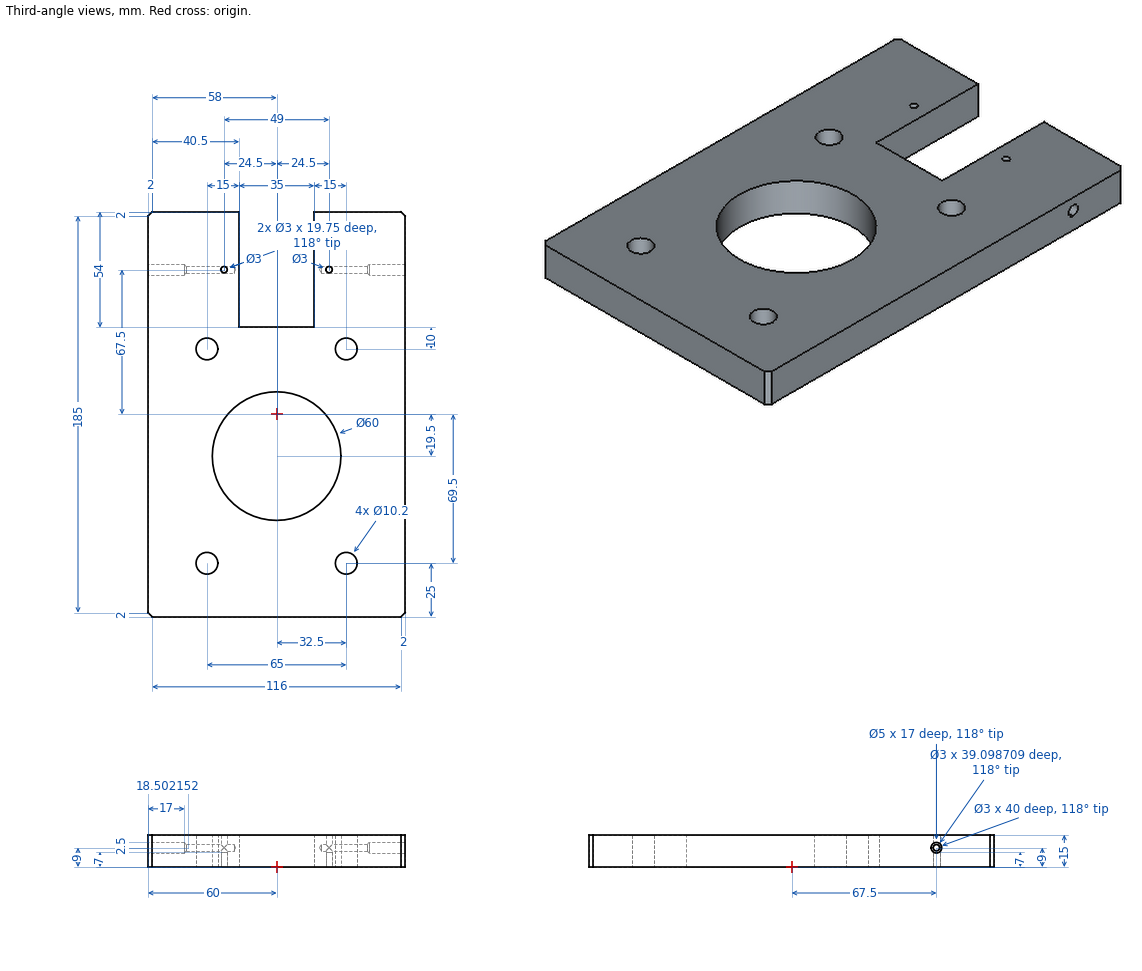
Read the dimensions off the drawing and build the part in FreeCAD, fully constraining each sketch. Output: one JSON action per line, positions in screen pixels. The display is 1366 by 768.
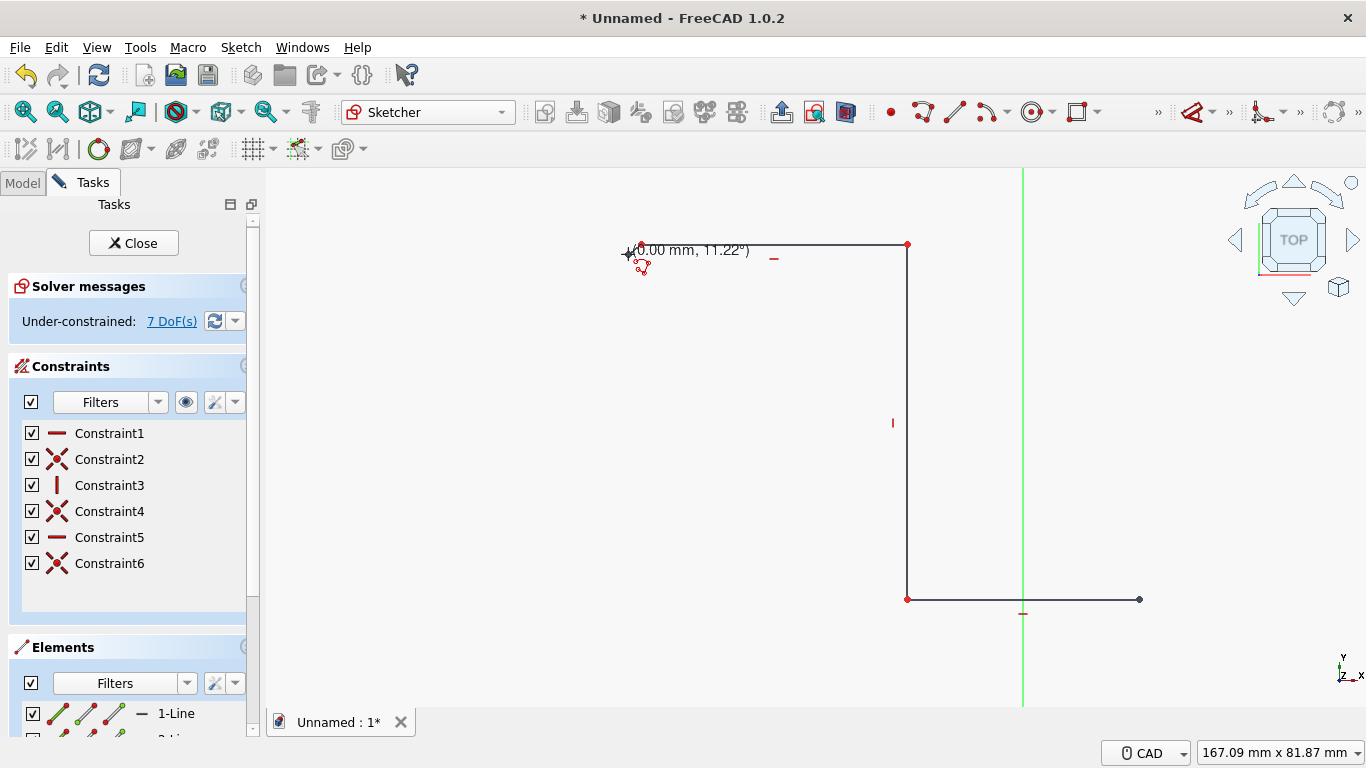
{"action": "scroll", "coordinate": [629, 254], "scroll_direction": "down", "scroll_amount": 6}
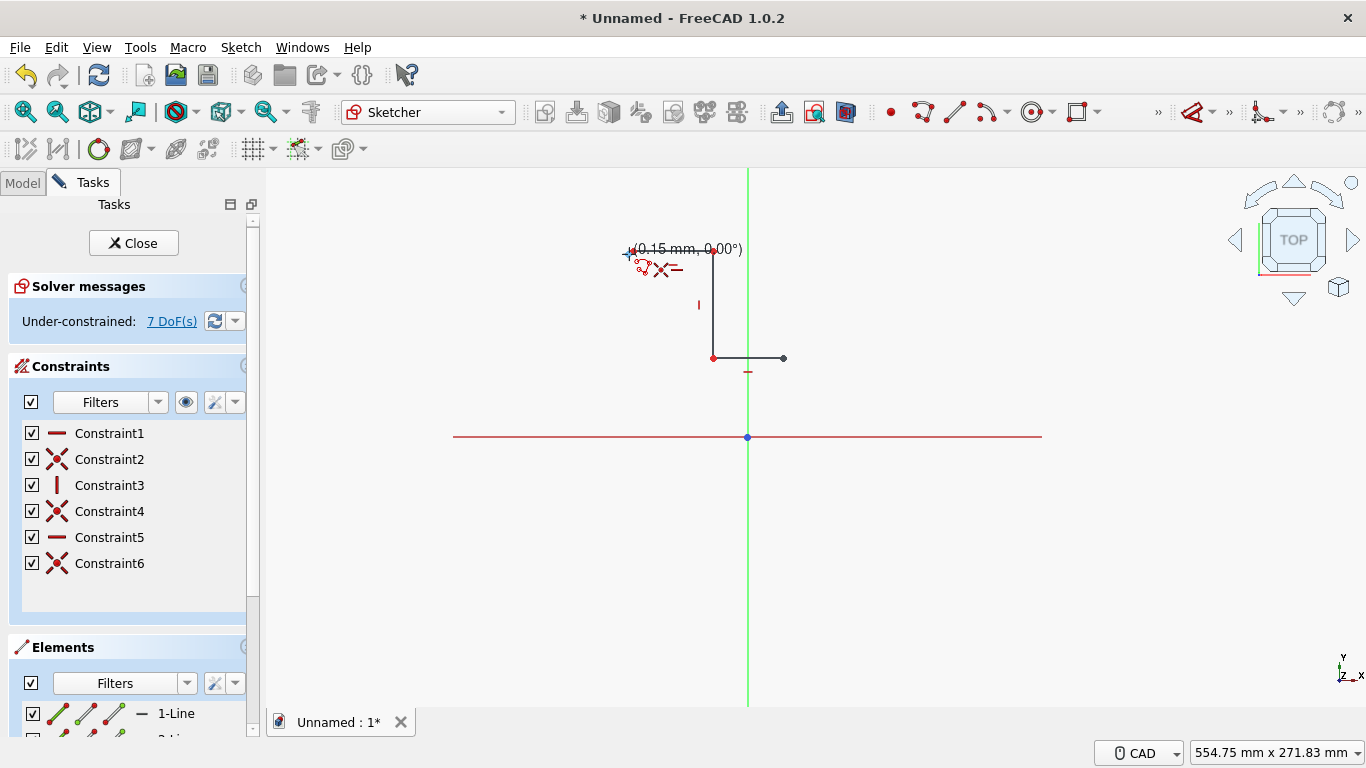
{"action": "left_click", "coordinate": [629, 621]}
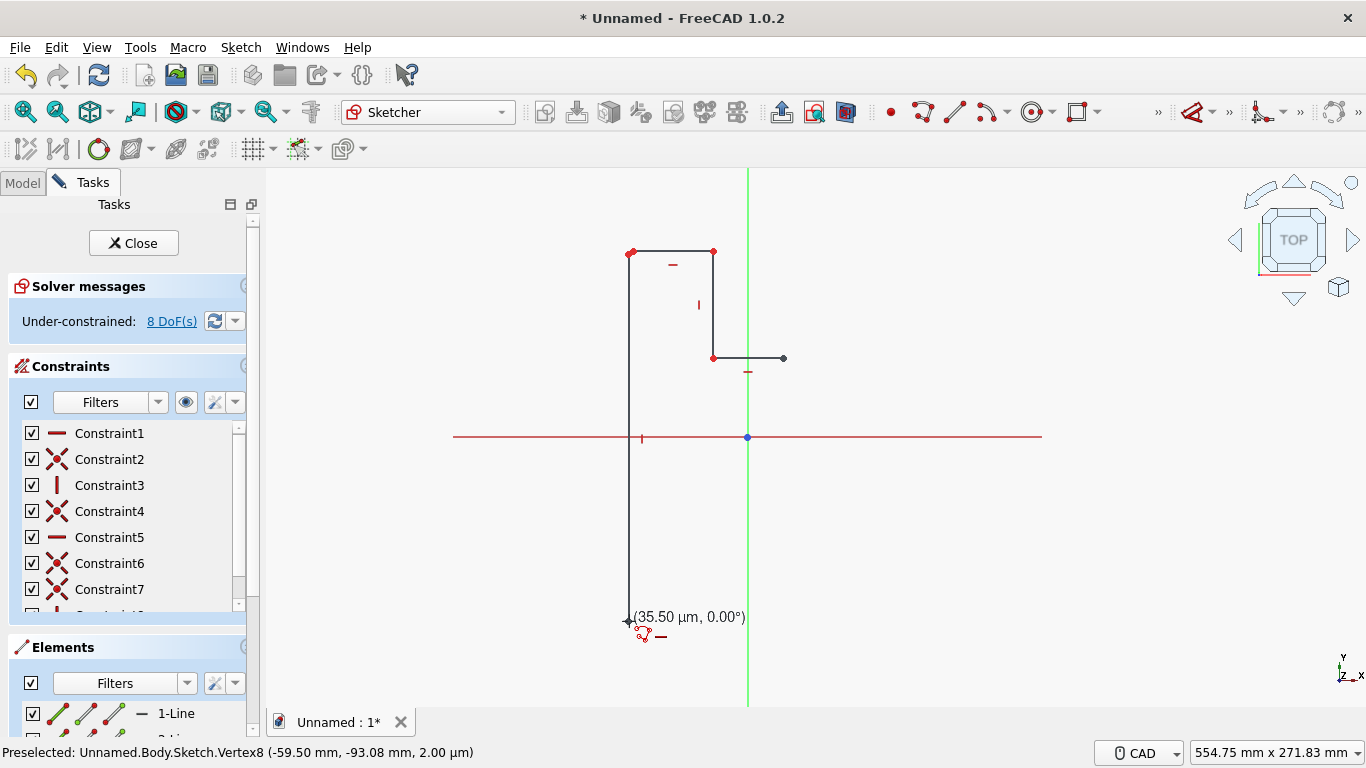
{"action": "scroll", "coordinate": [633, 625], "scroll_direction": "up", "scroll_amount": 6}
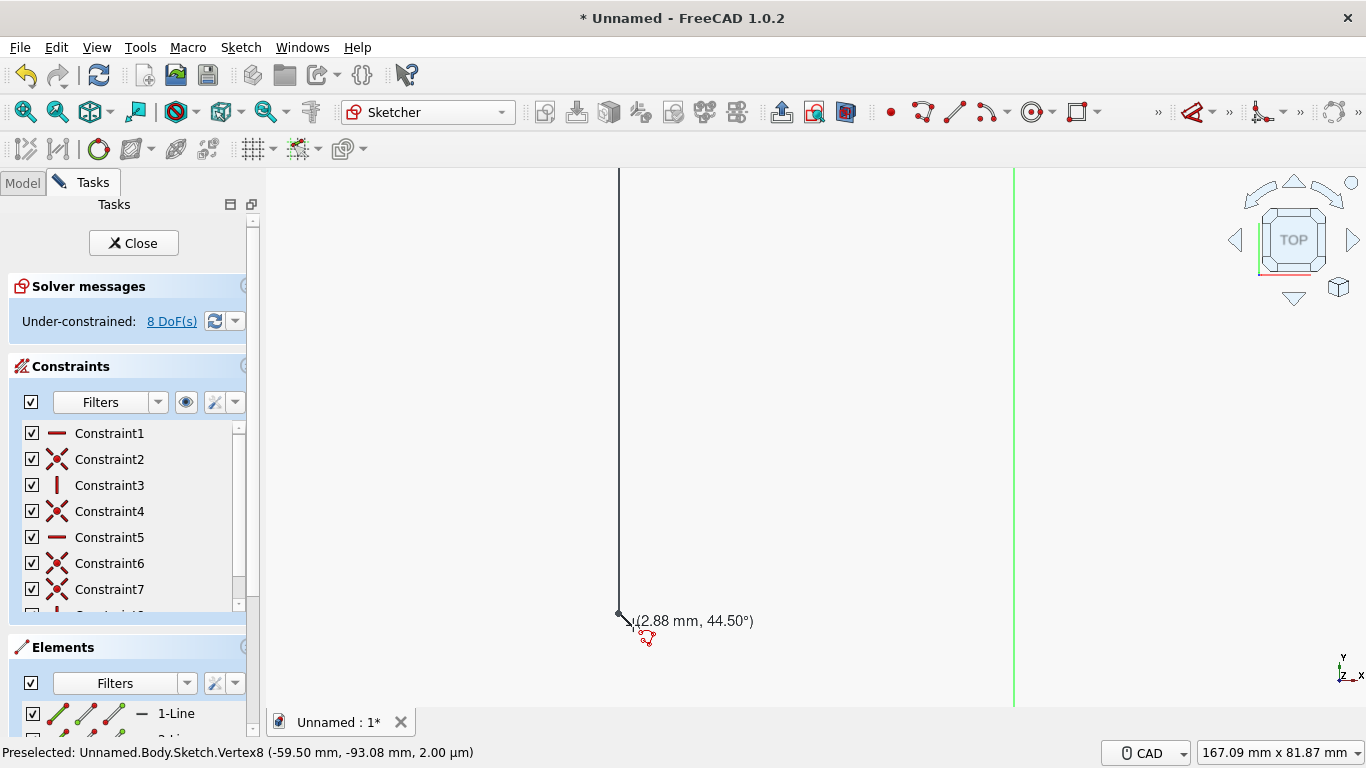
{"action": "left_click", "coordinate": [632, 622]}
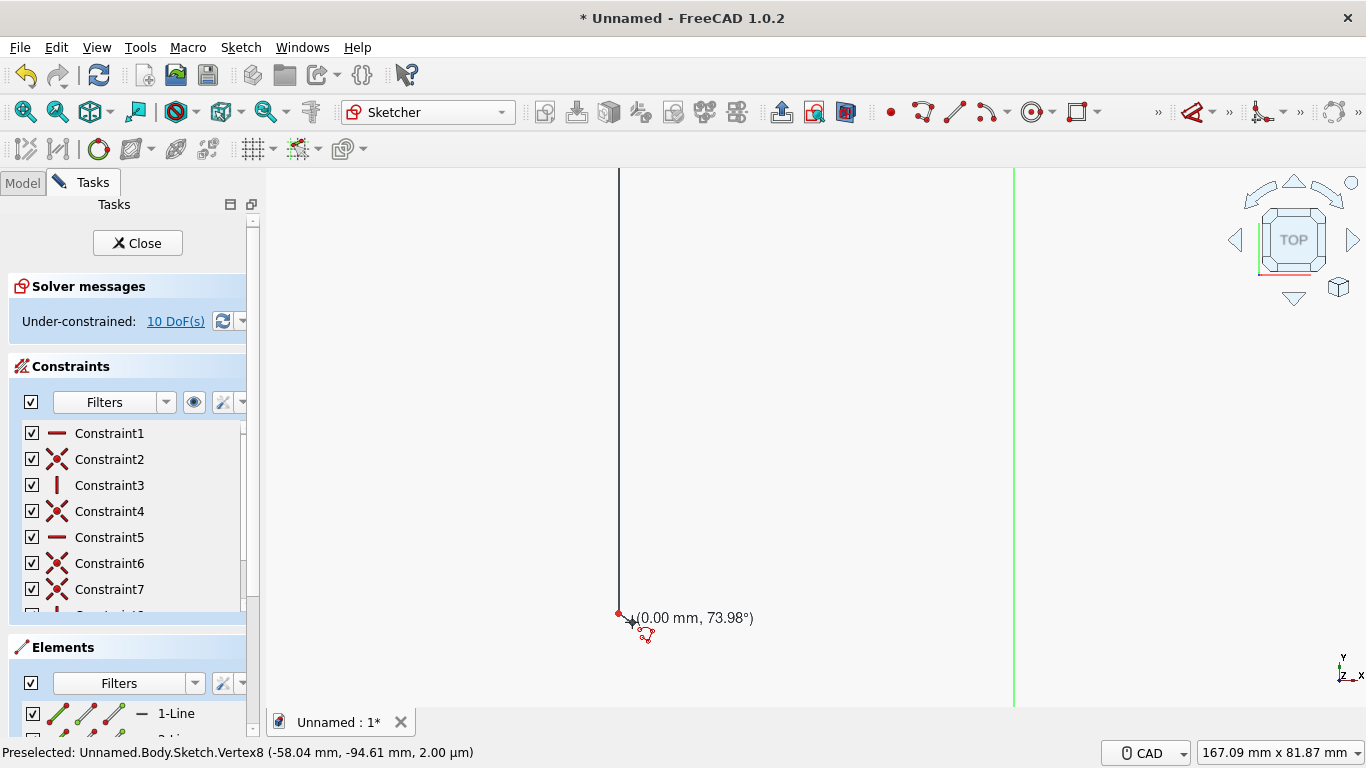
{"action": "scroll", "coordinate": [633, 626], "scroll_direction": "down", "scroll_amount": 6}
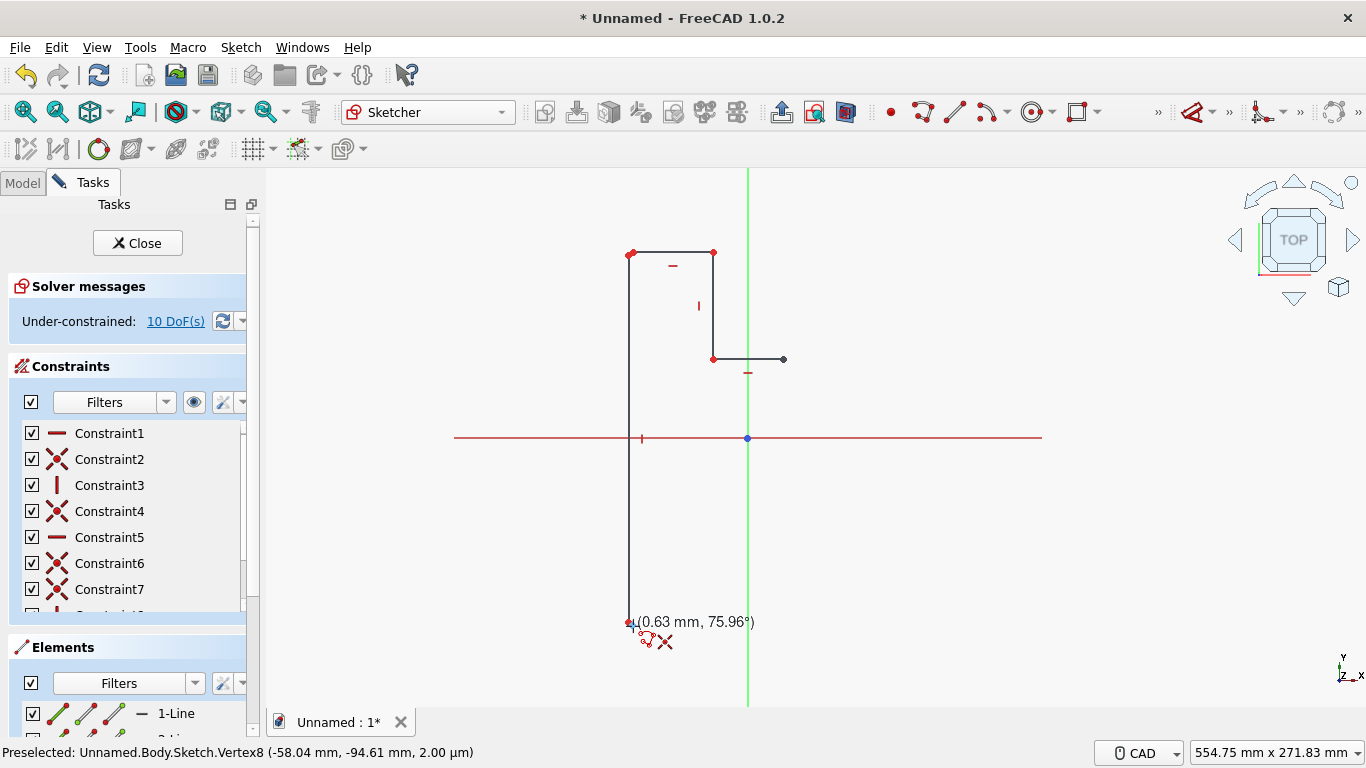
{"action": "left_click", "coordinate": [863, 625]}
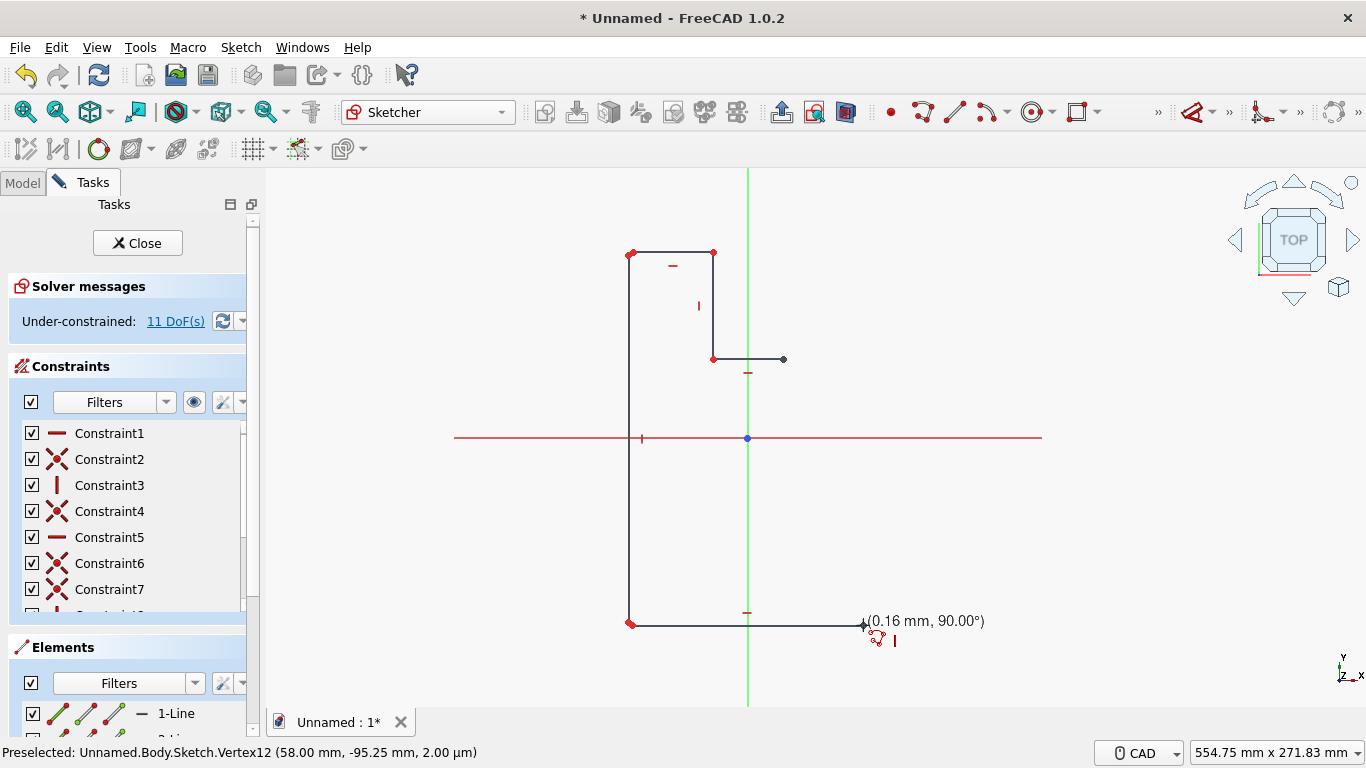
{"action": "scroll", "coordinate": [867, 622], "scroll_direction": "up", "scroll_amount": 6}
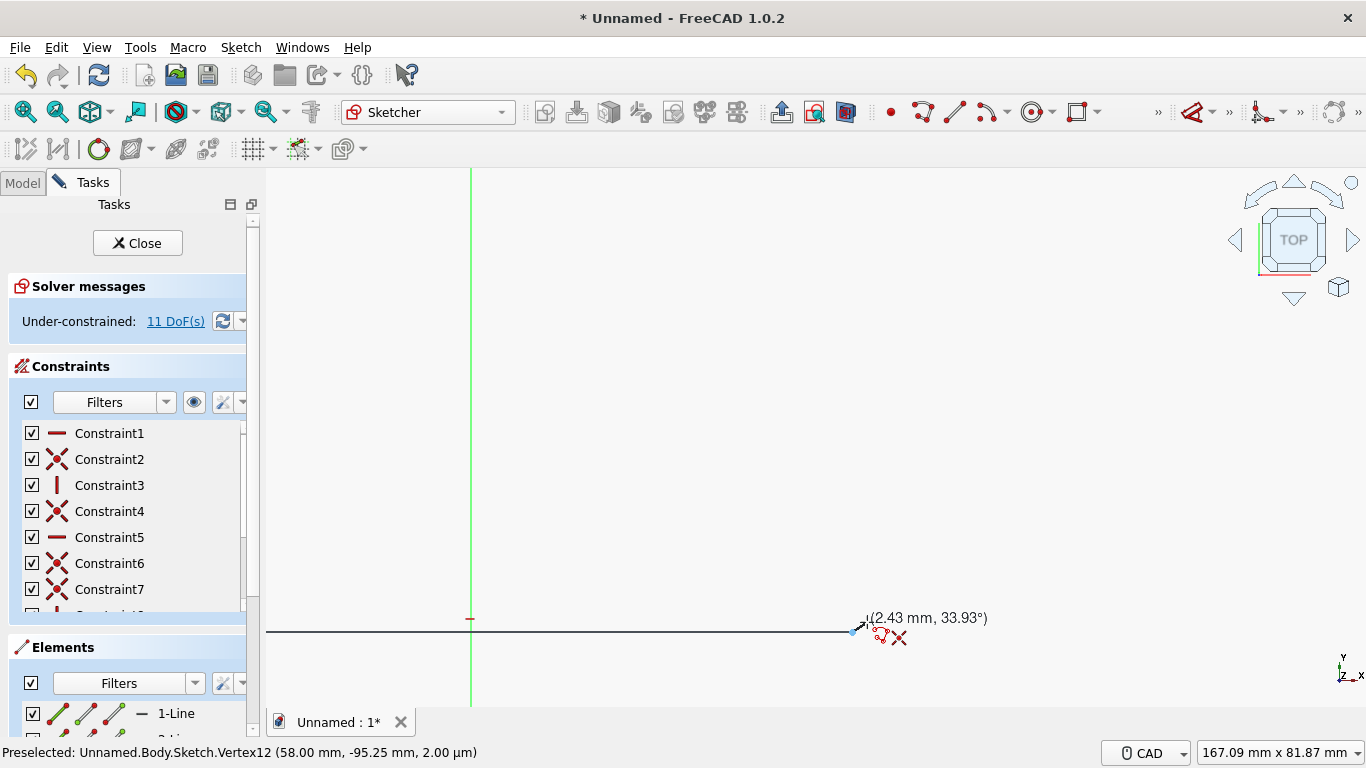
{"action": "left_click", "coordinate": [866, 619]}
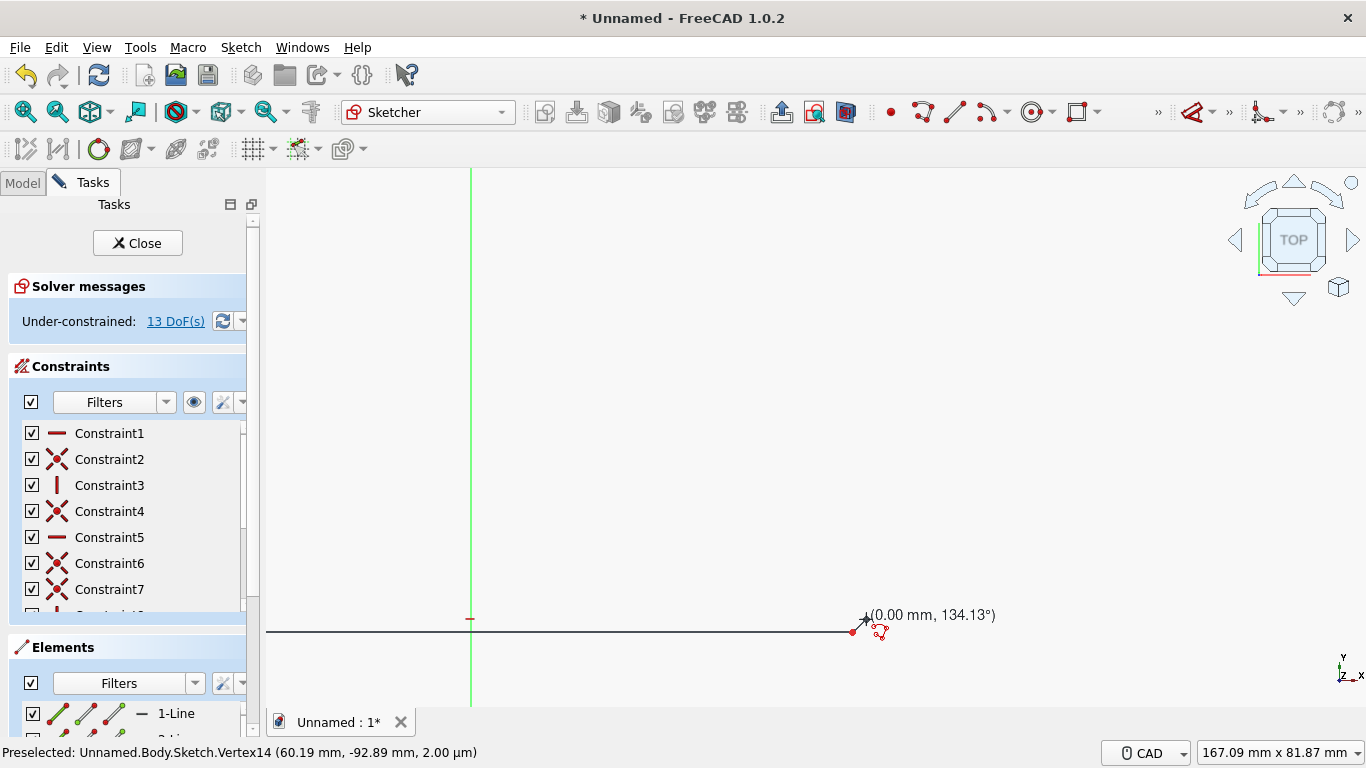
{"action": "scroll", "coordinate": [867, 622], "scroll_direction": "down", "scroll_amount": 6}